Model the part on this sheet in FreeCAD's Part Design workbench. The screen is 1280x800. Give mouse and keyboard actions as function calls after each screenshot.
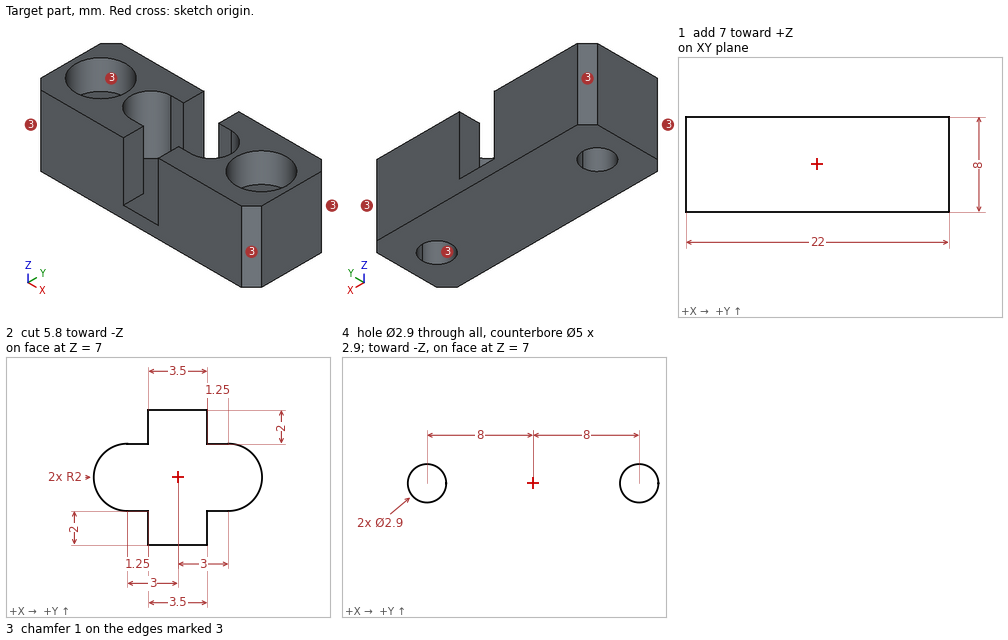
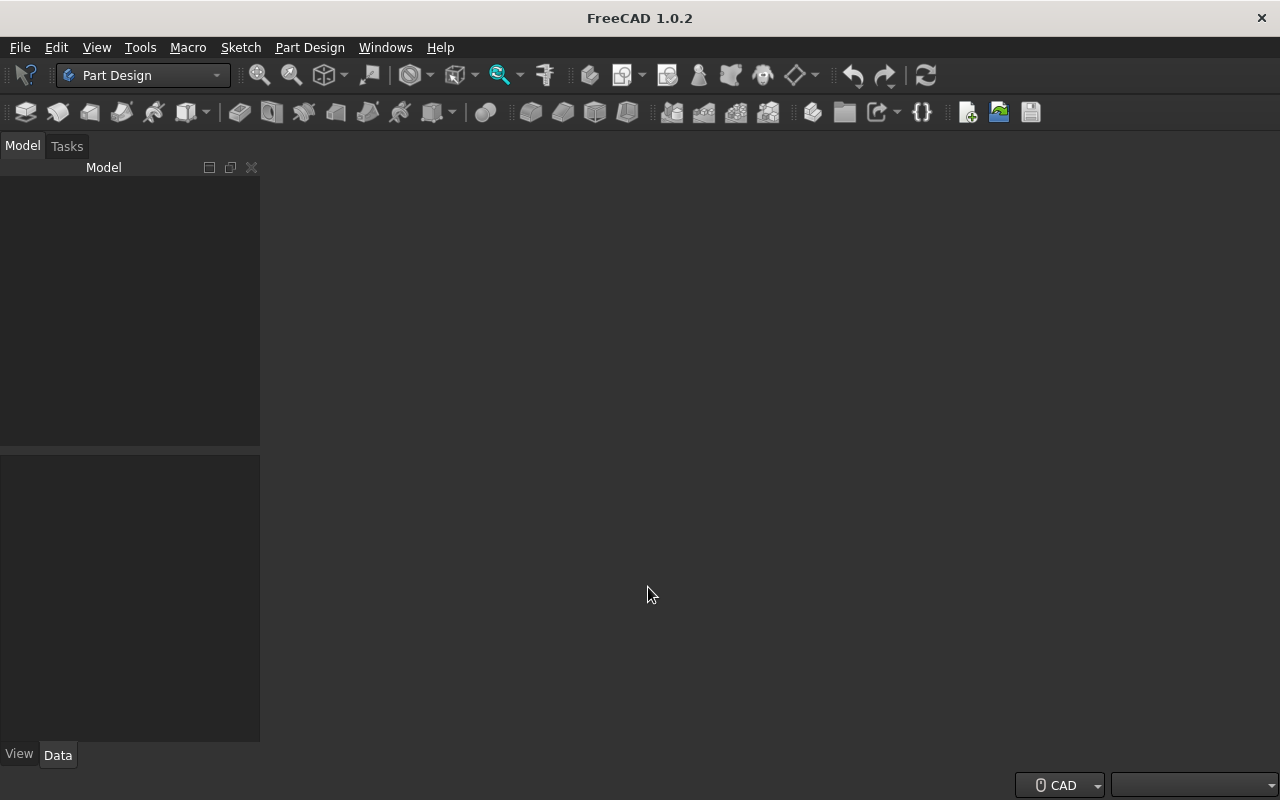
click(968, 112)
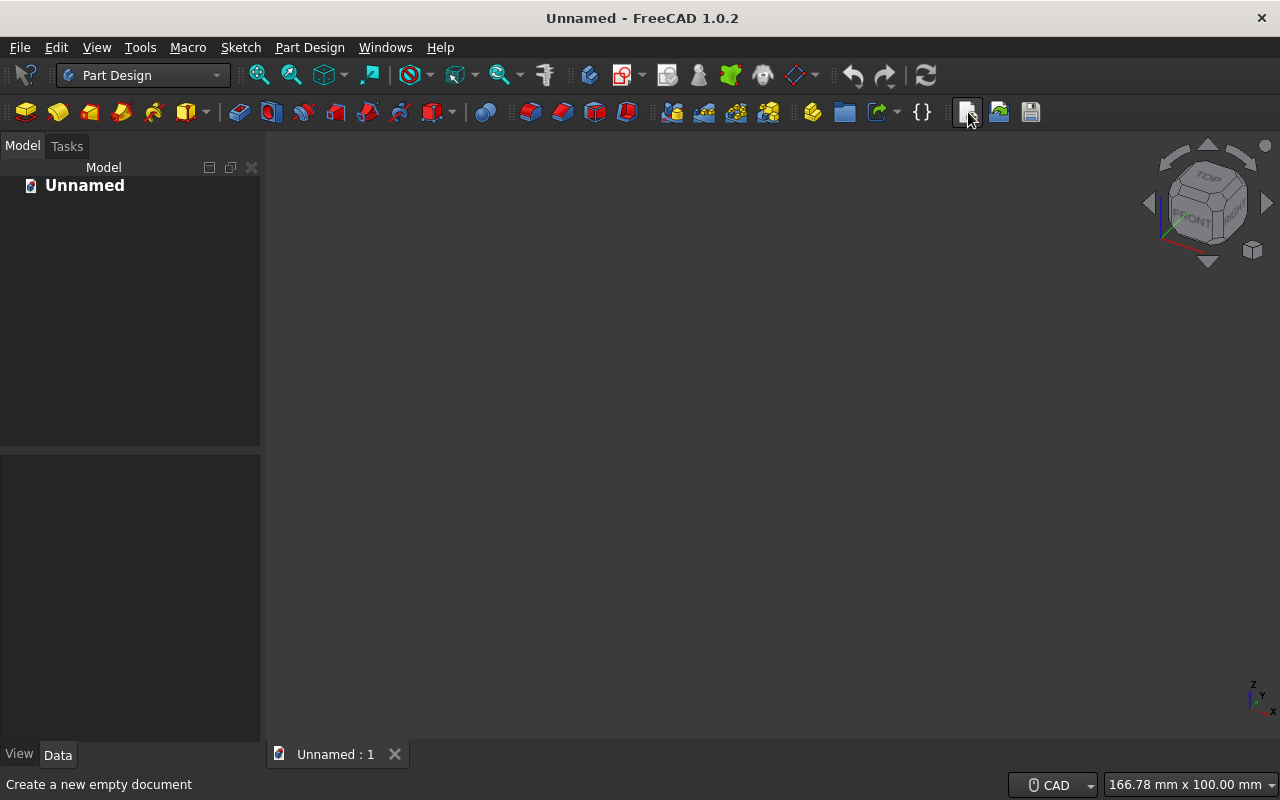
click(622, 76)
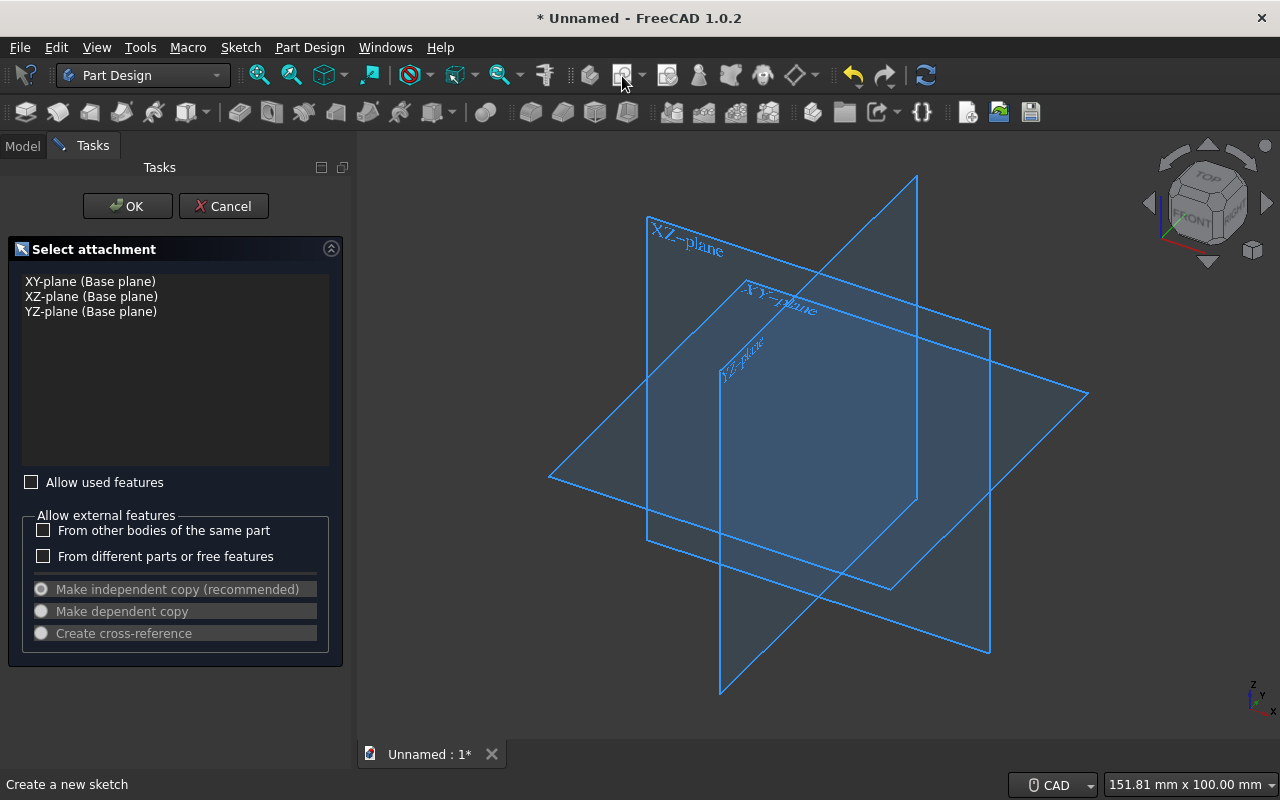
click(82, 282)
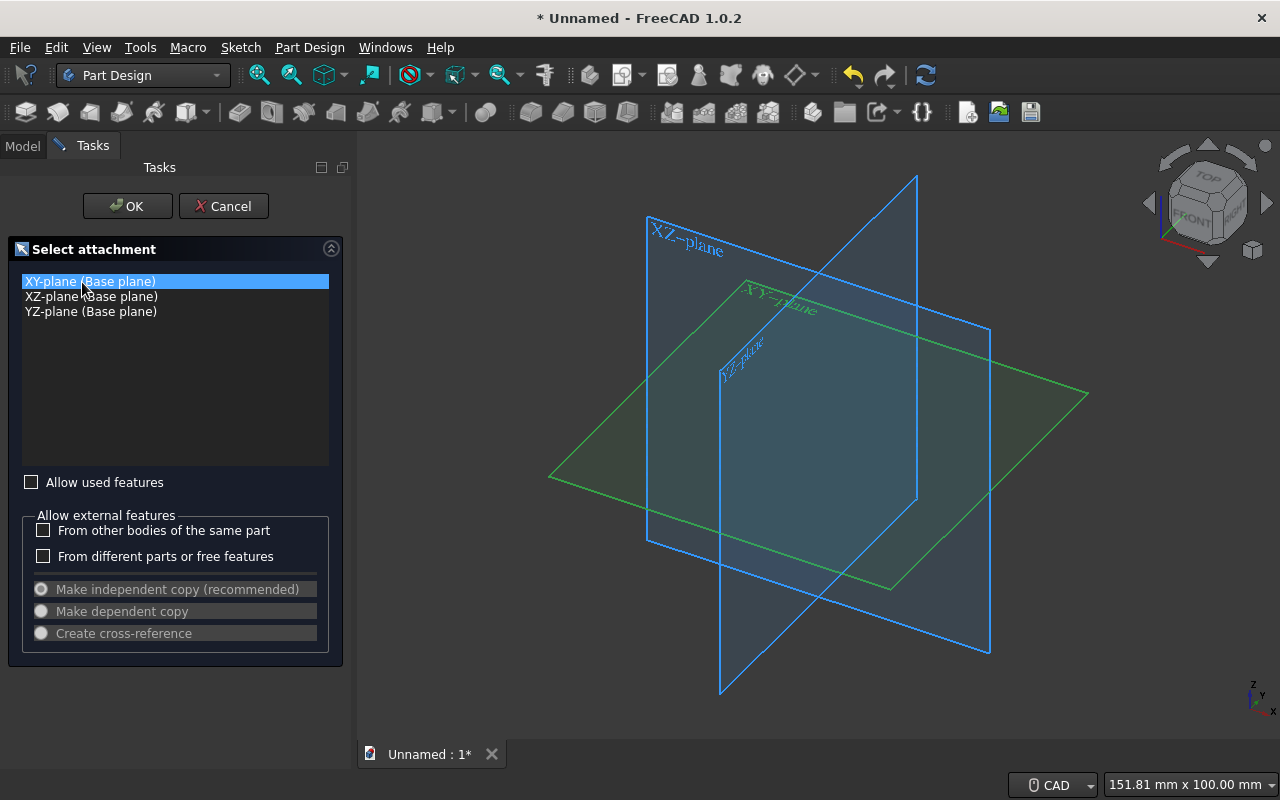
click(128, 206)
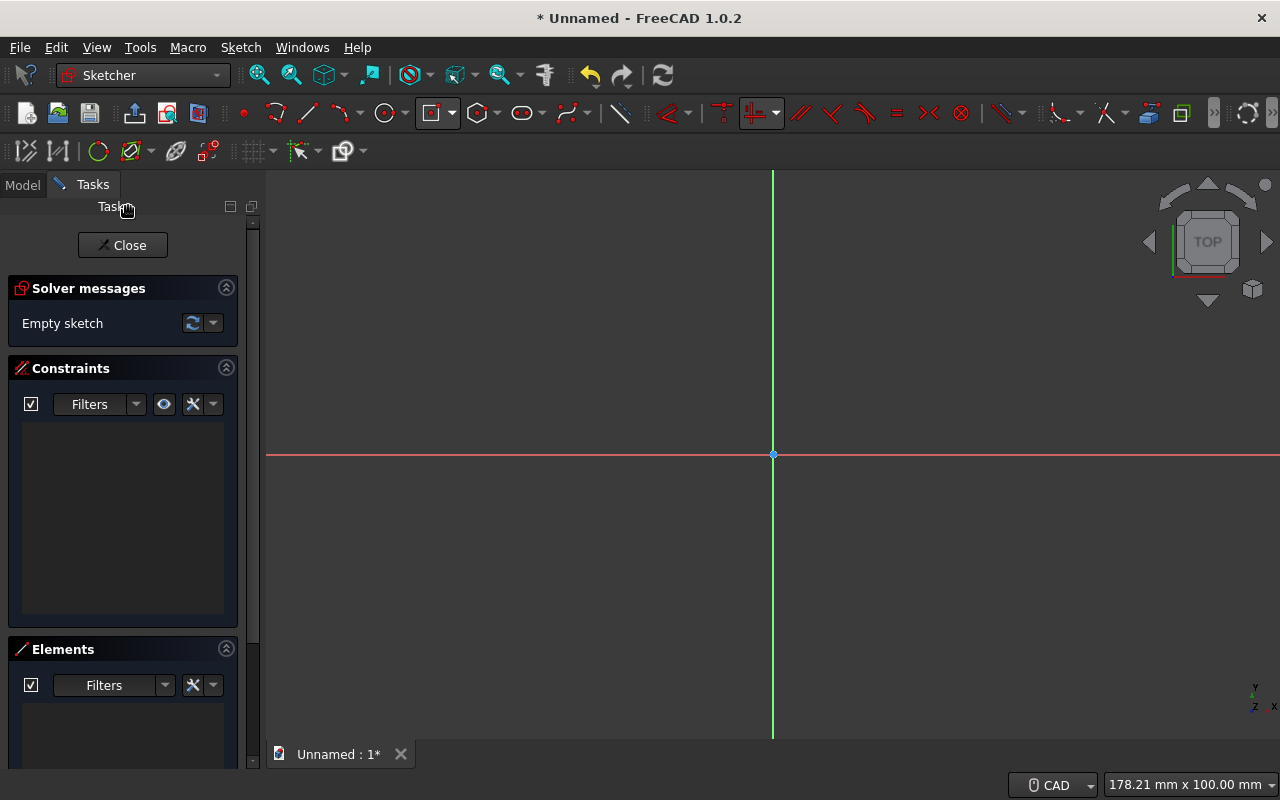
scroll(790, 454, up, 8)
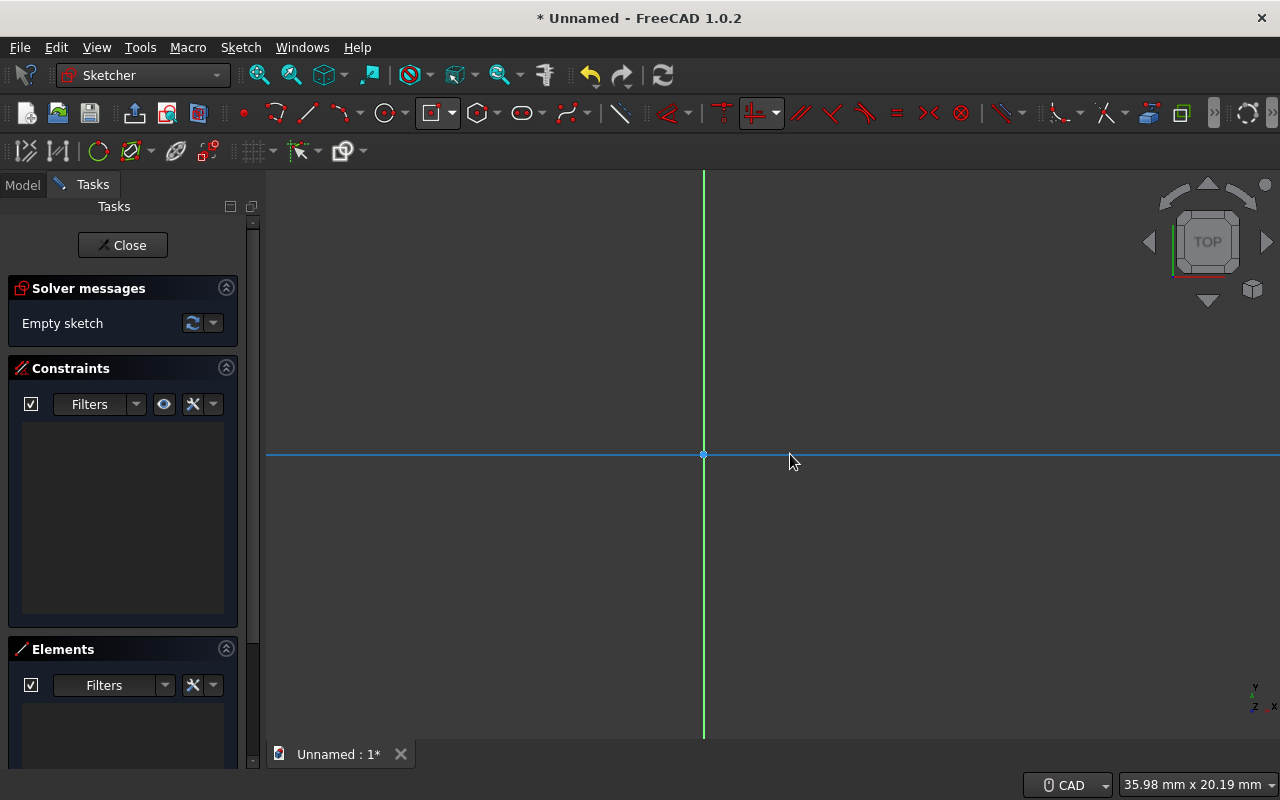
click(432, 114)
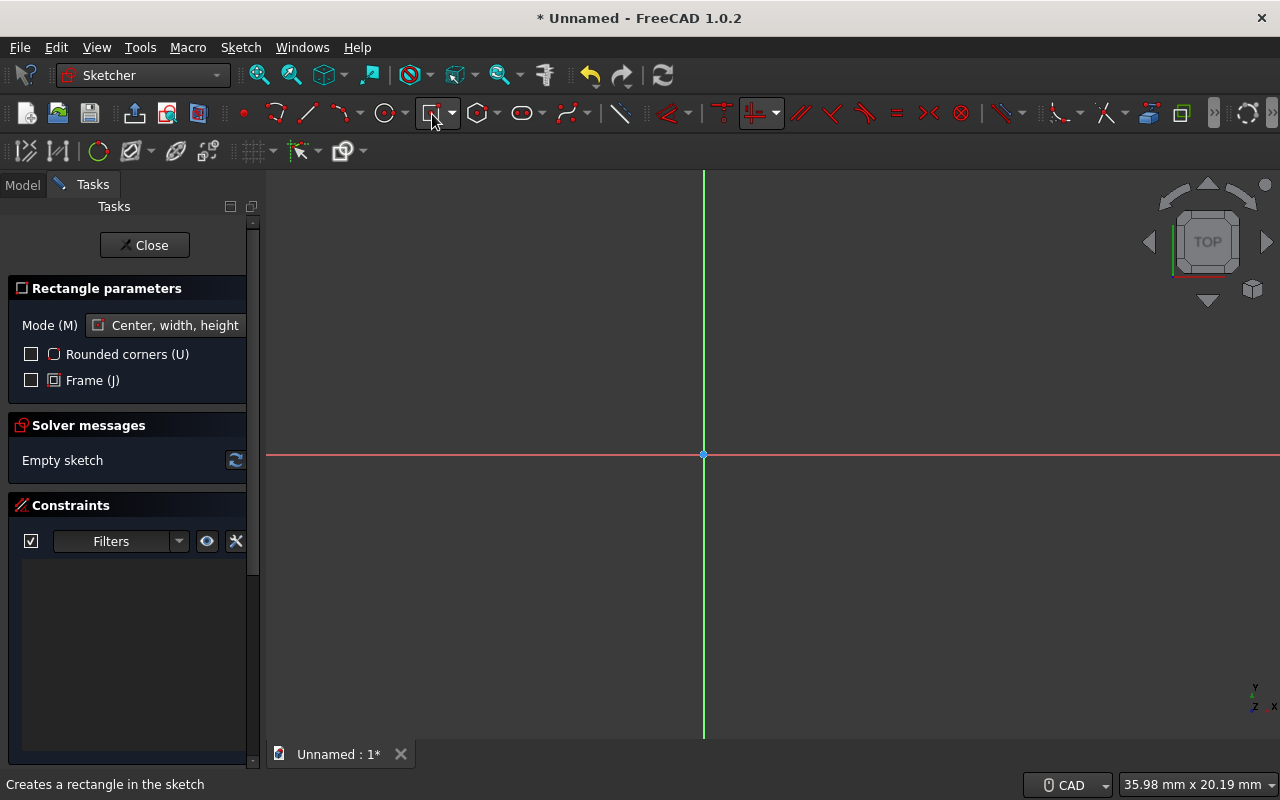
click(704, 454)
click(1014, 342)
key(Escape)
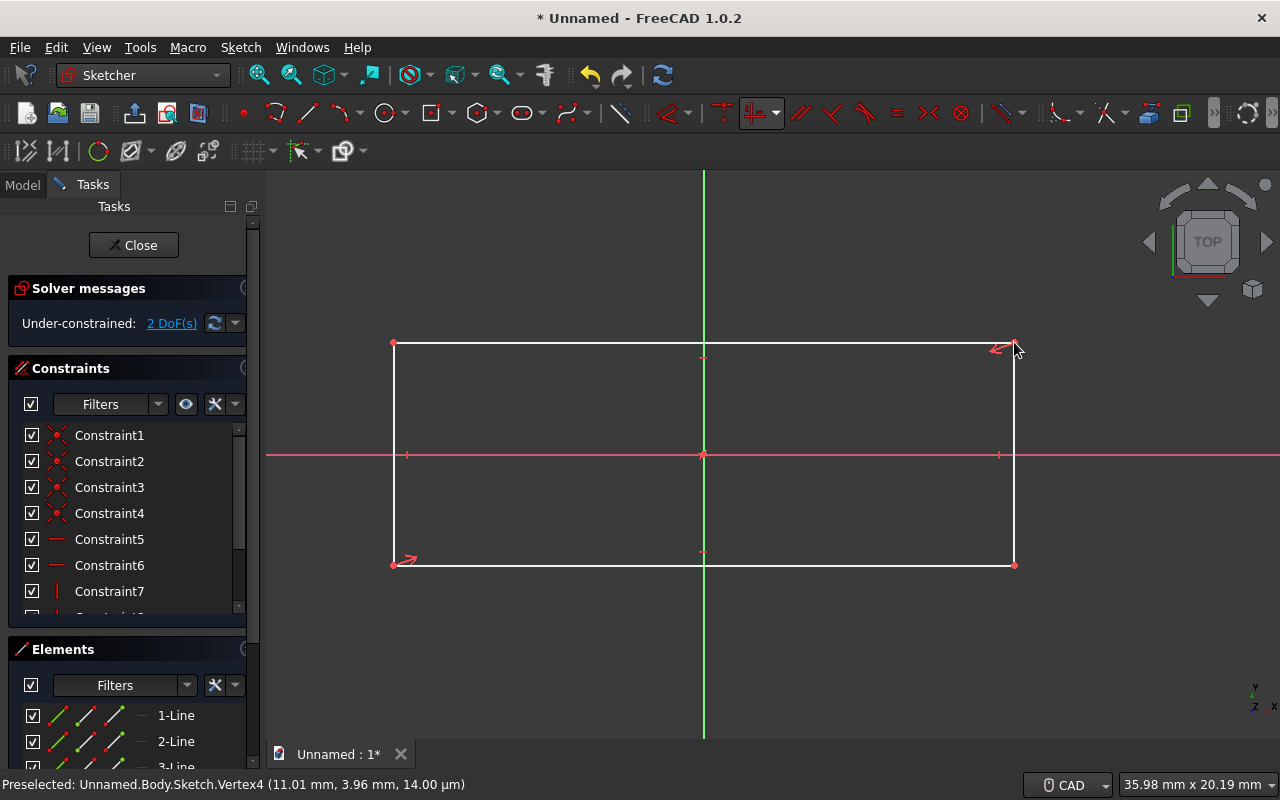
click(1014, 499)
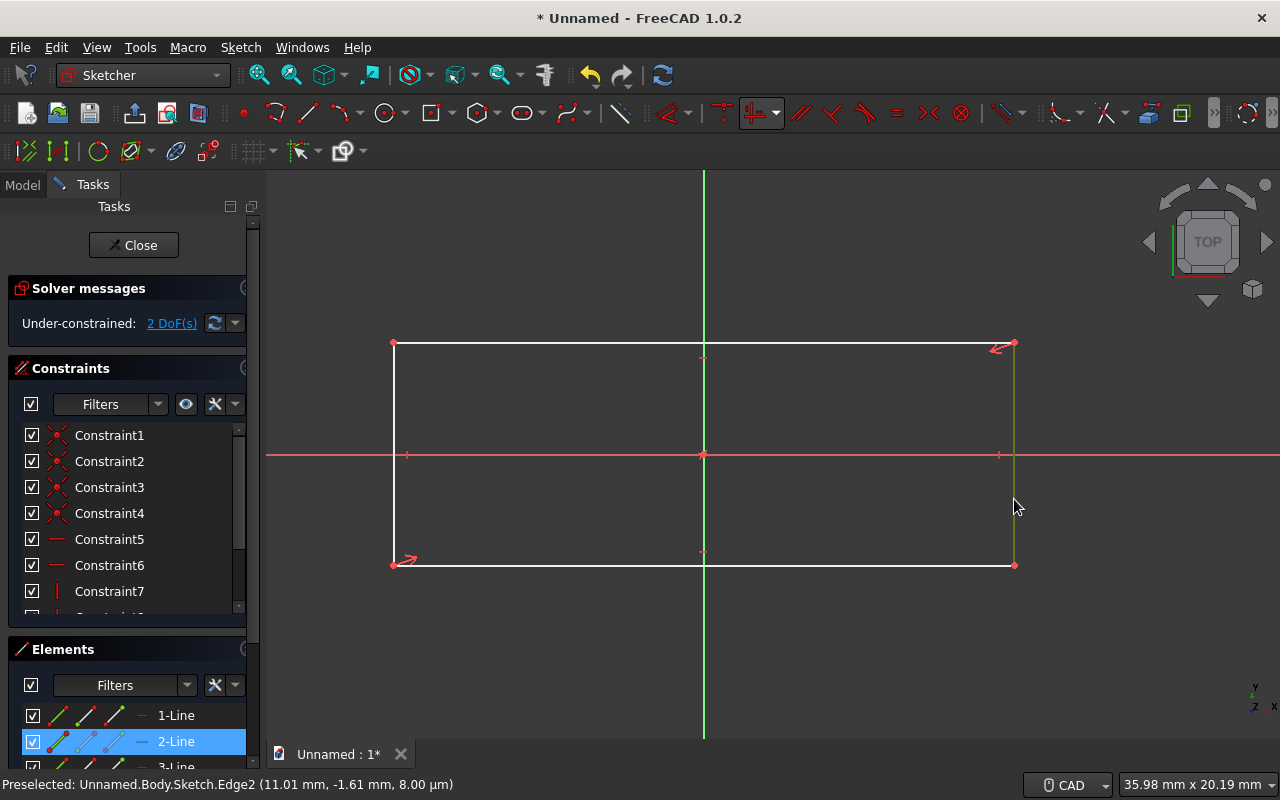
key(i)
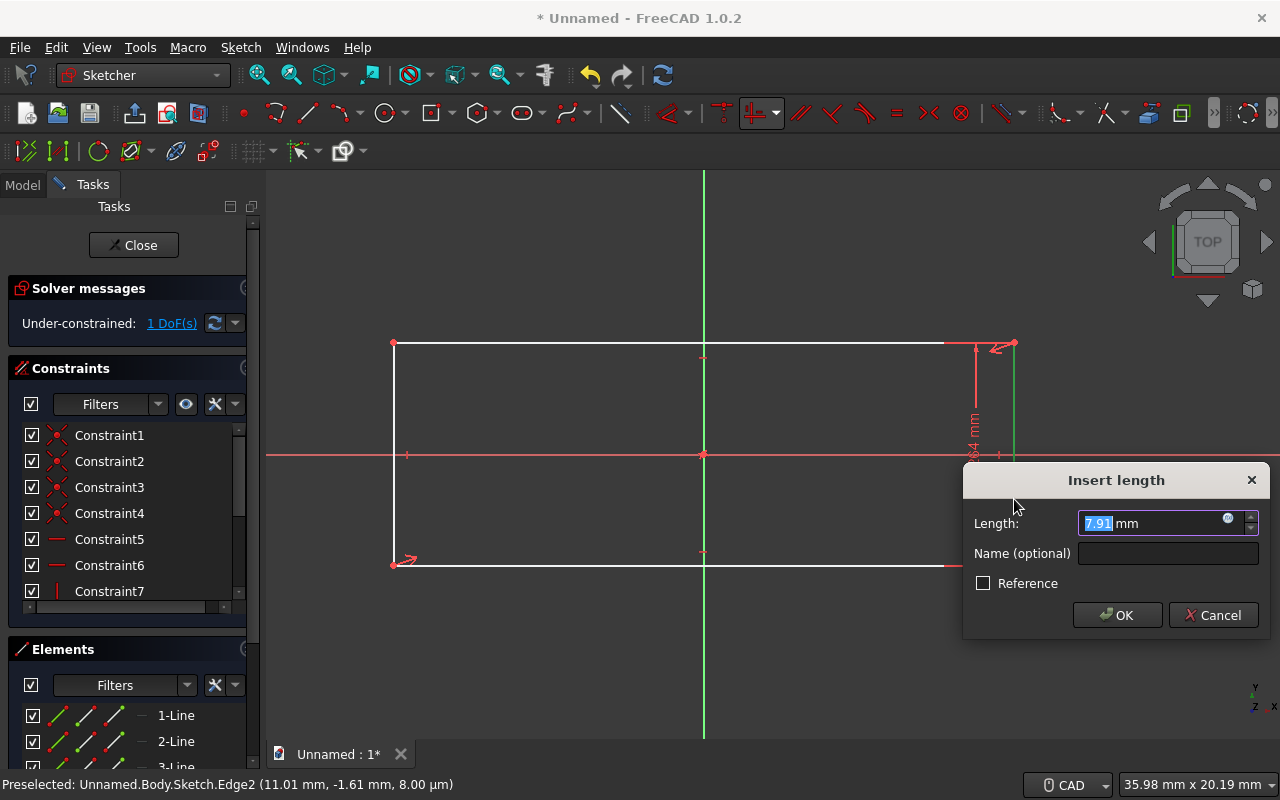
text(8)
key(Return)